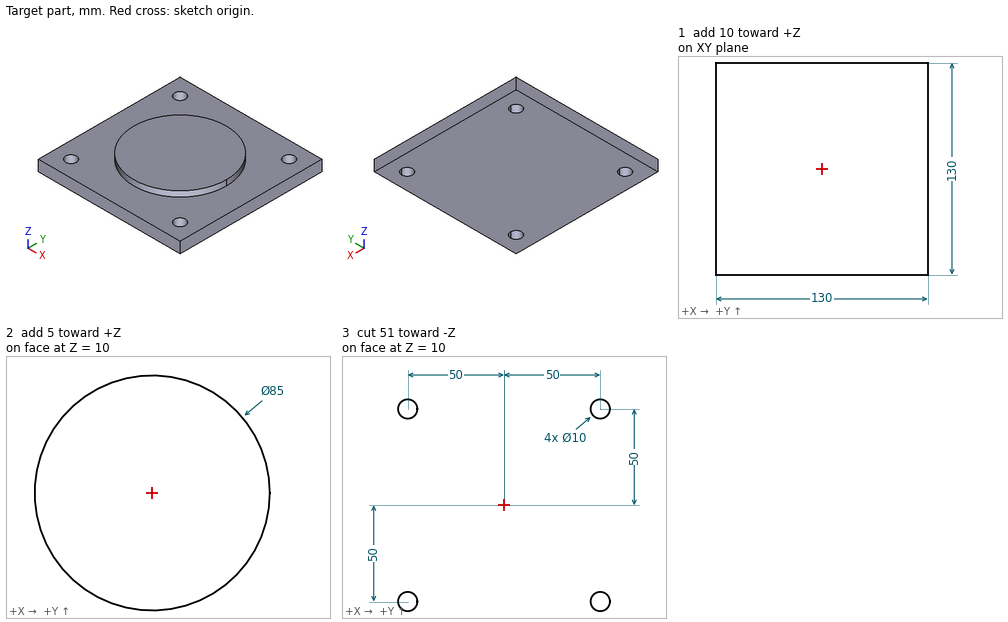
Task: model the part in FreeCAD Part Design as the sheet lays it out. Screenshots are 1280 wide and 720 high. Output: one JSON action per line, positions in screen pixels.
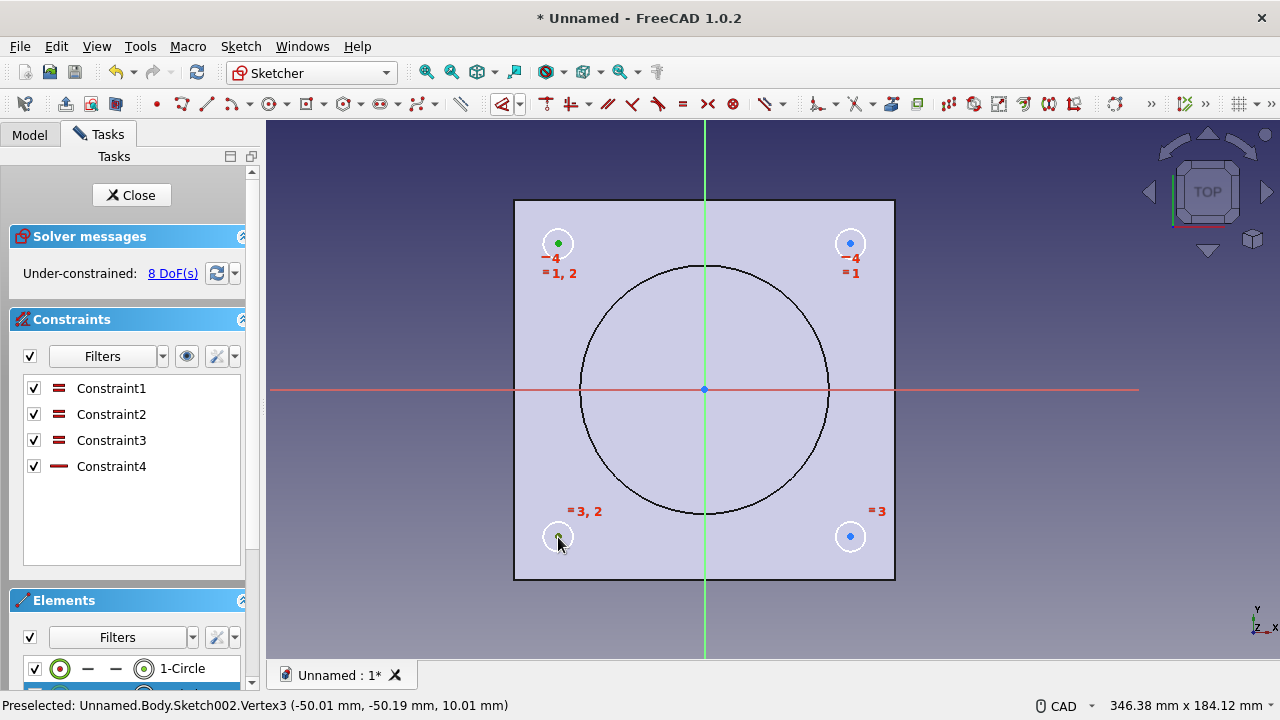
{"action": "key", "text": "v"}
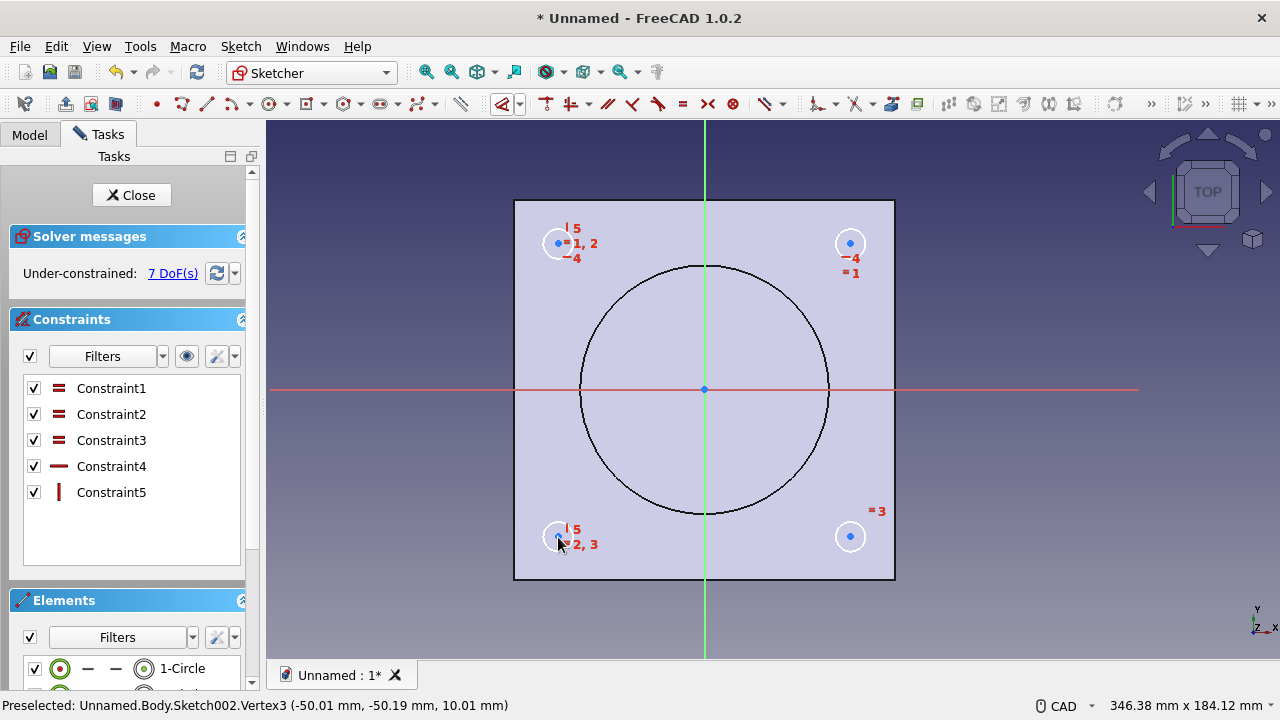
{"action": "left_click", "coordinate": [851, 244]}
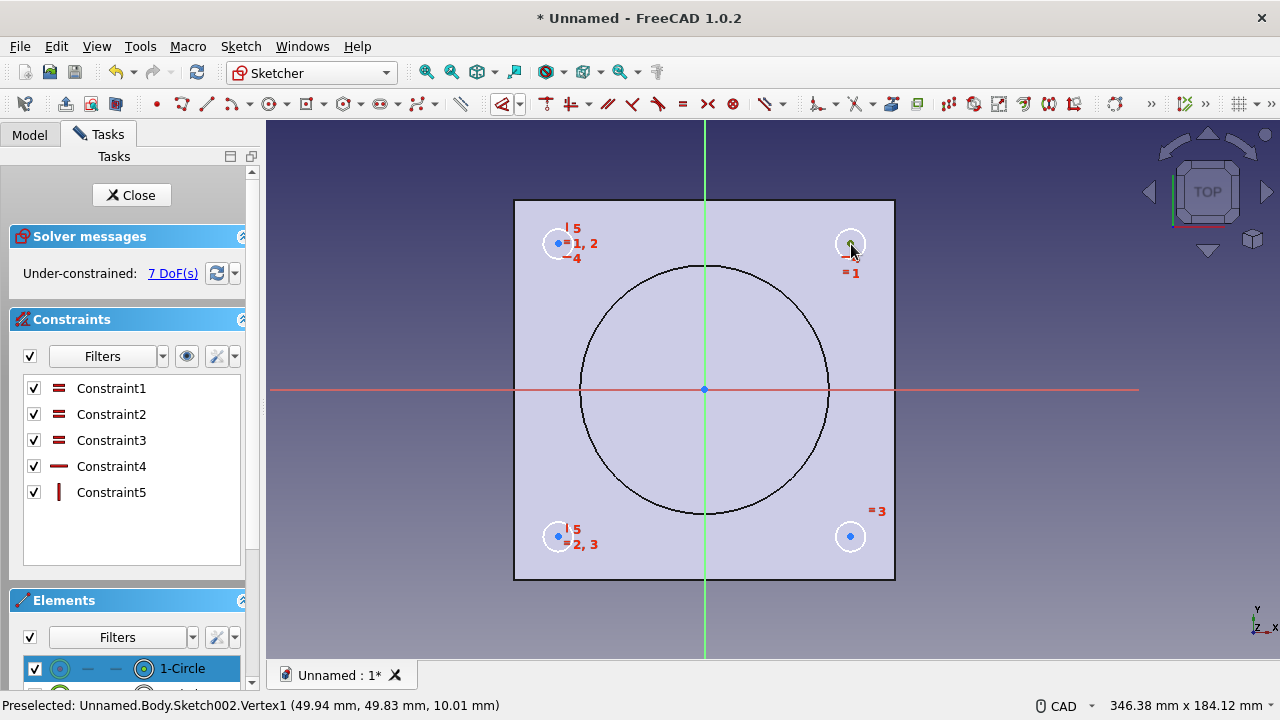
{"action": "left_click", "coordinate": [851, 537]}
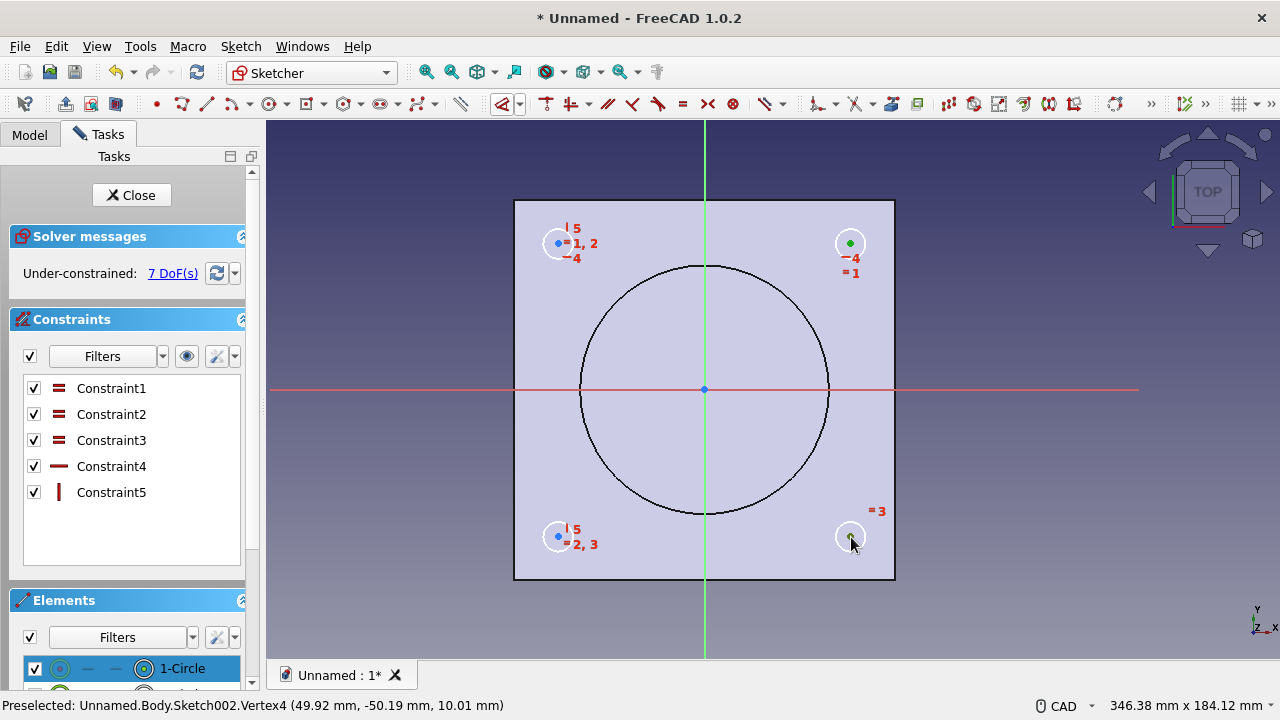
{"action": "left_click", "coordinate": [588, 104]}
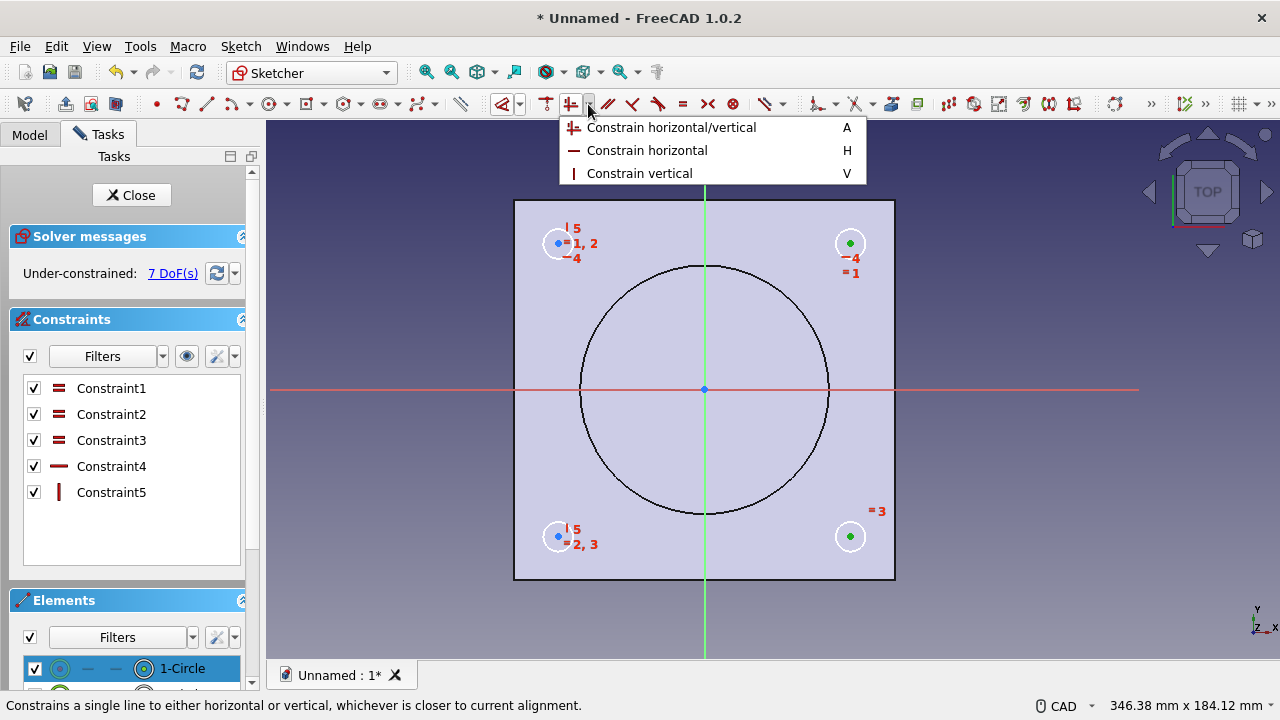
{"action": "left_click", "coordinate": [713, 174]}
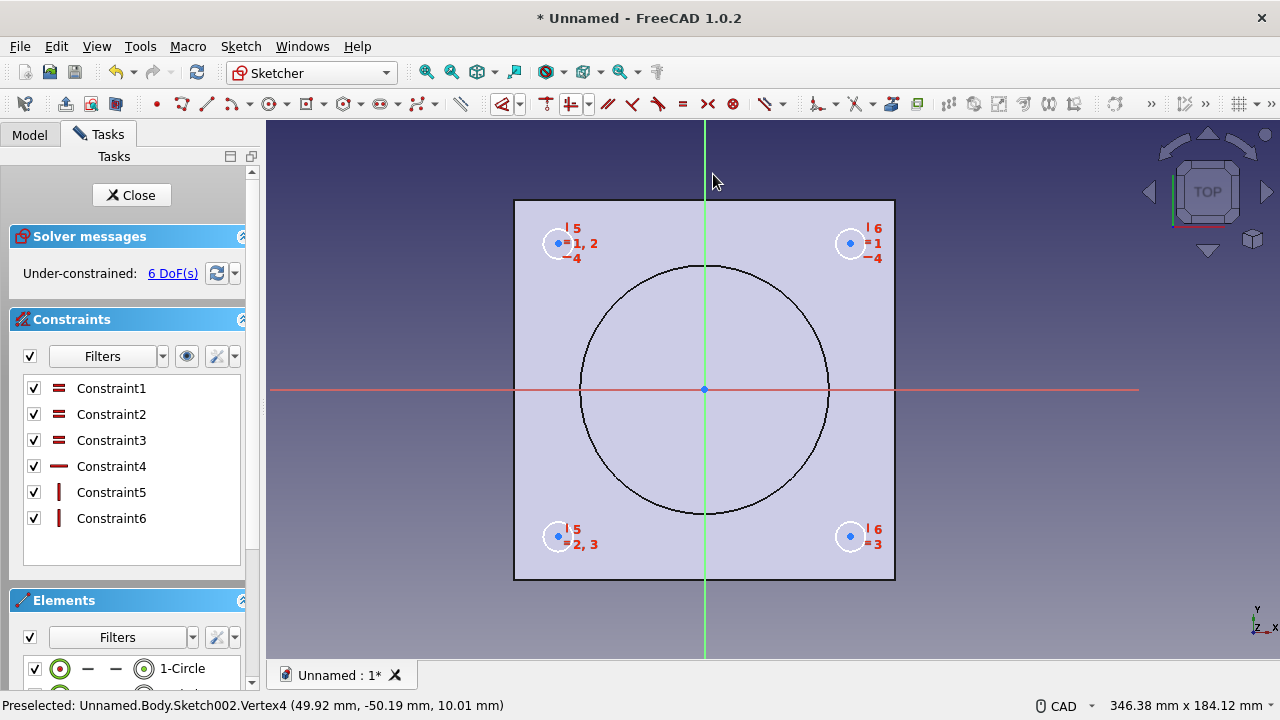
{"action": "left_click", "coordinate": [558, 537]}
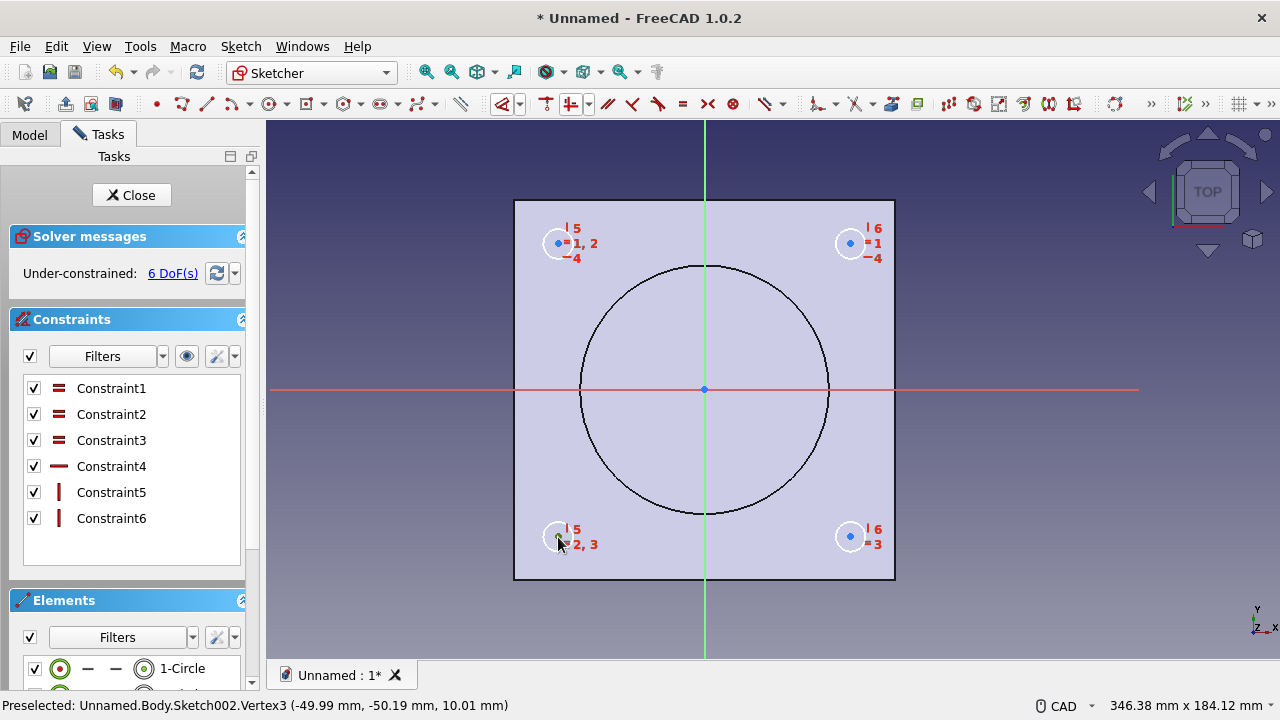
{"action": "left_click", "coordinate": [851, 537]}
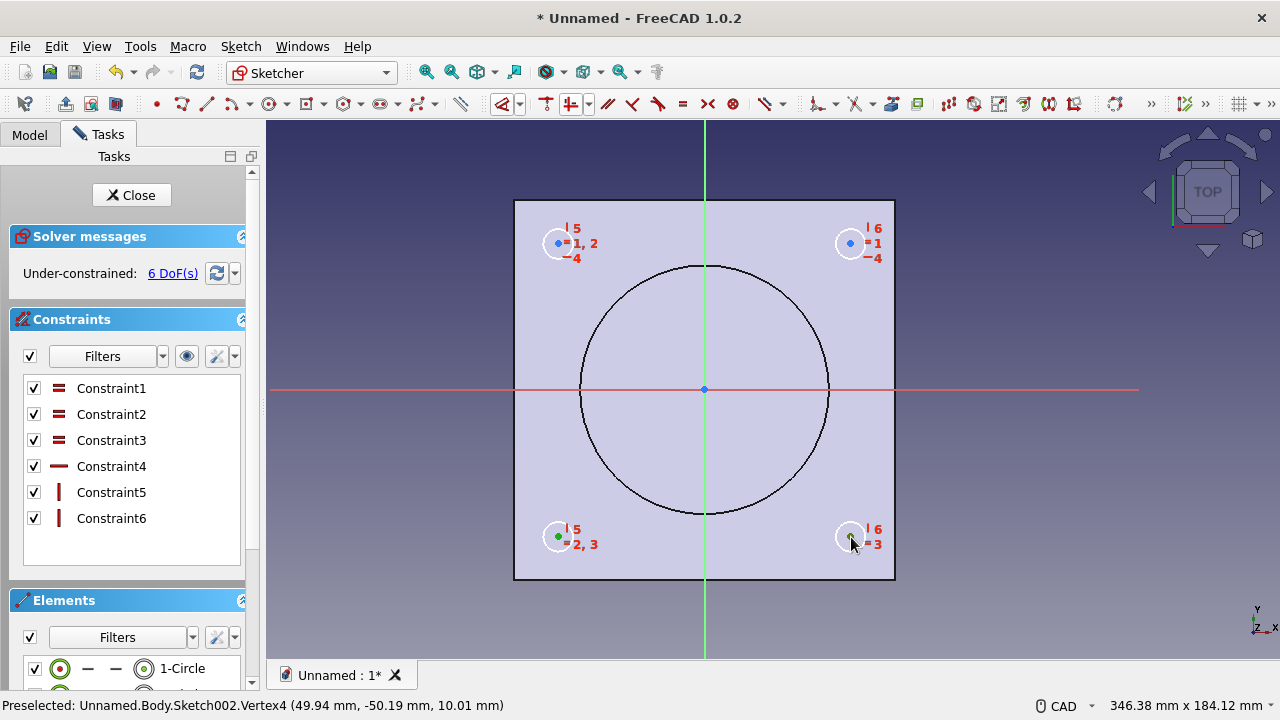
{"action": "key", "text": "h"}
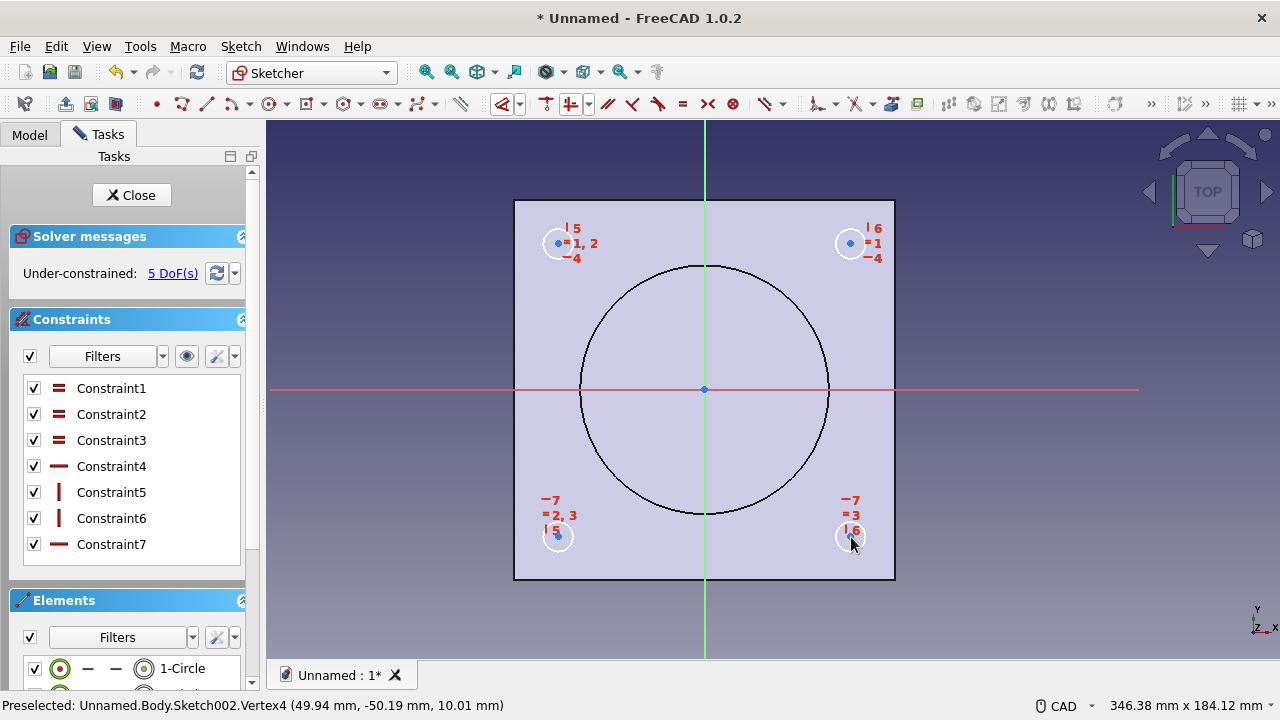
{"action": "scroll", "coordinate": [861, 234], "scroll_direction": "up", "scroll_amount": 2}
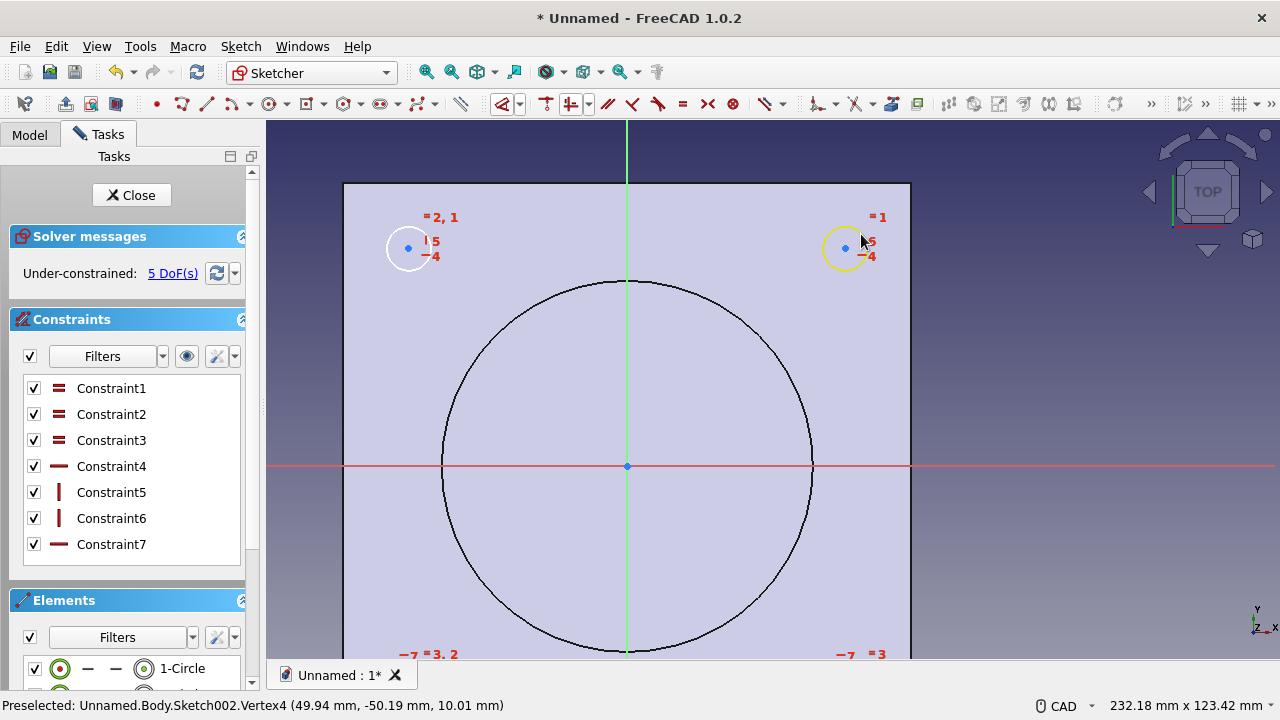
{"action": "left_click", "coordinate": [830, 233]}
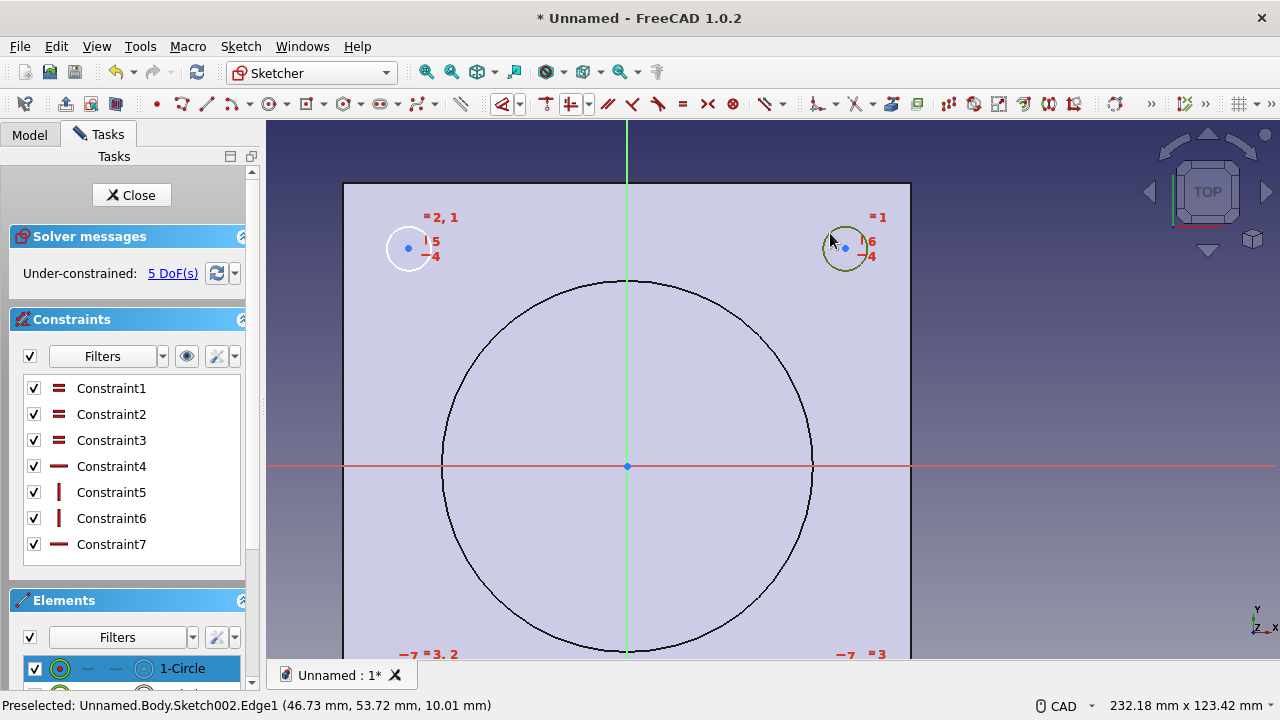
{"action": "key", "text": "k o"}